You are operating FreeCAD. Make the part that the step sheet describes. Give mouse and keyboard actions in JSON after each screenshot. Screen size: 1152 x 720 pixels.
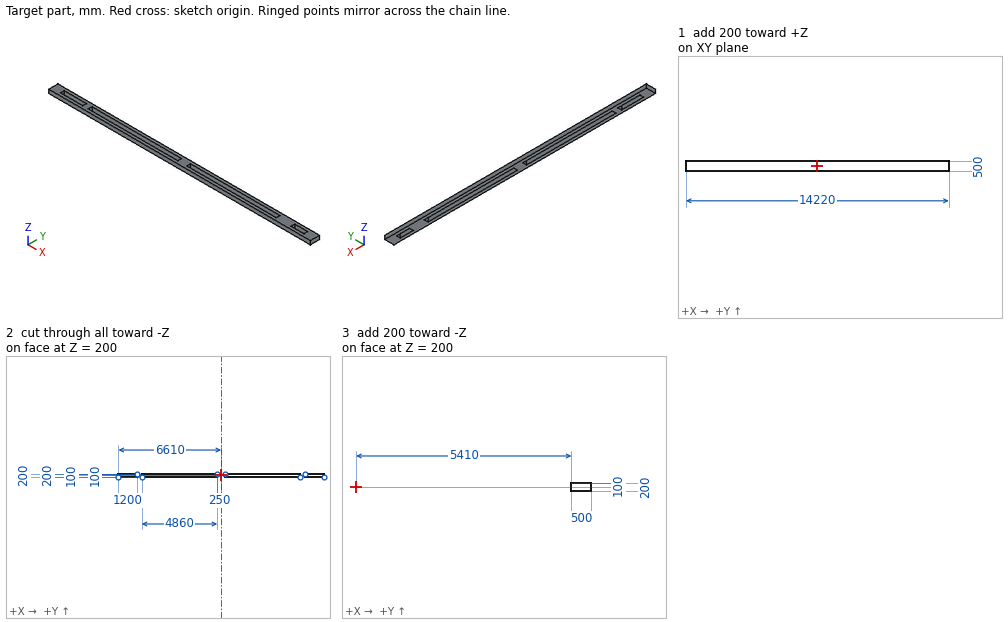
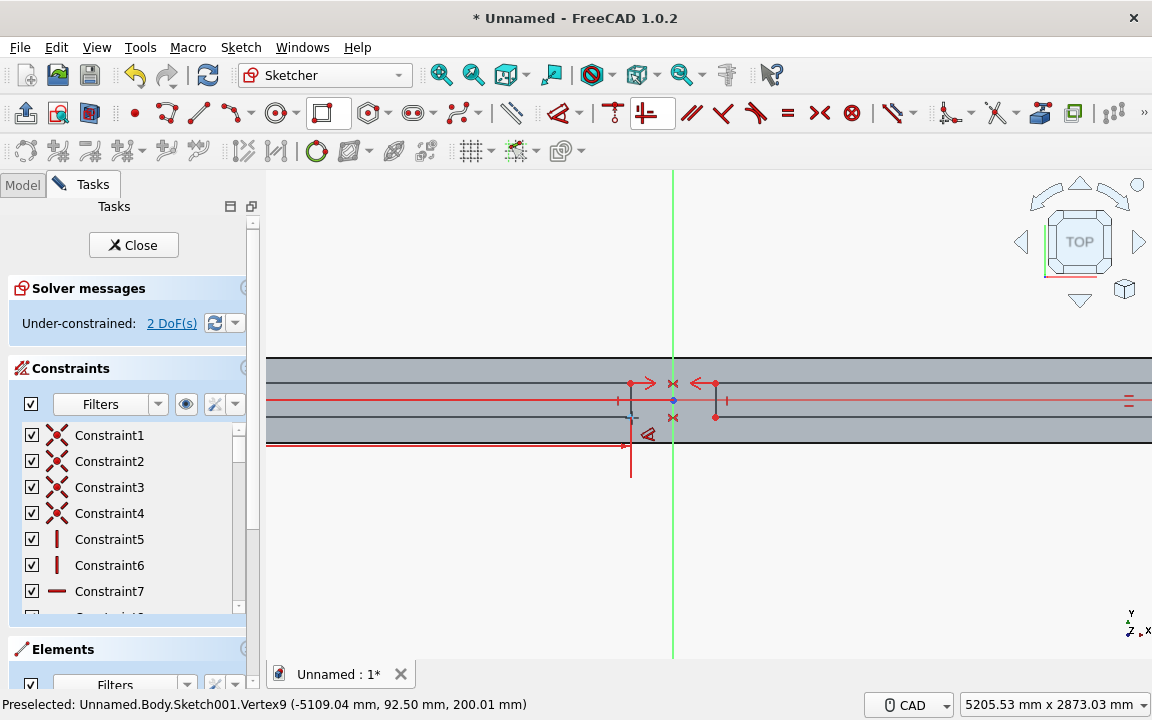
{"action": "left_click", "coordinate": [631, 417]}
{"action": "left_click", "coordinate": [652, 451]}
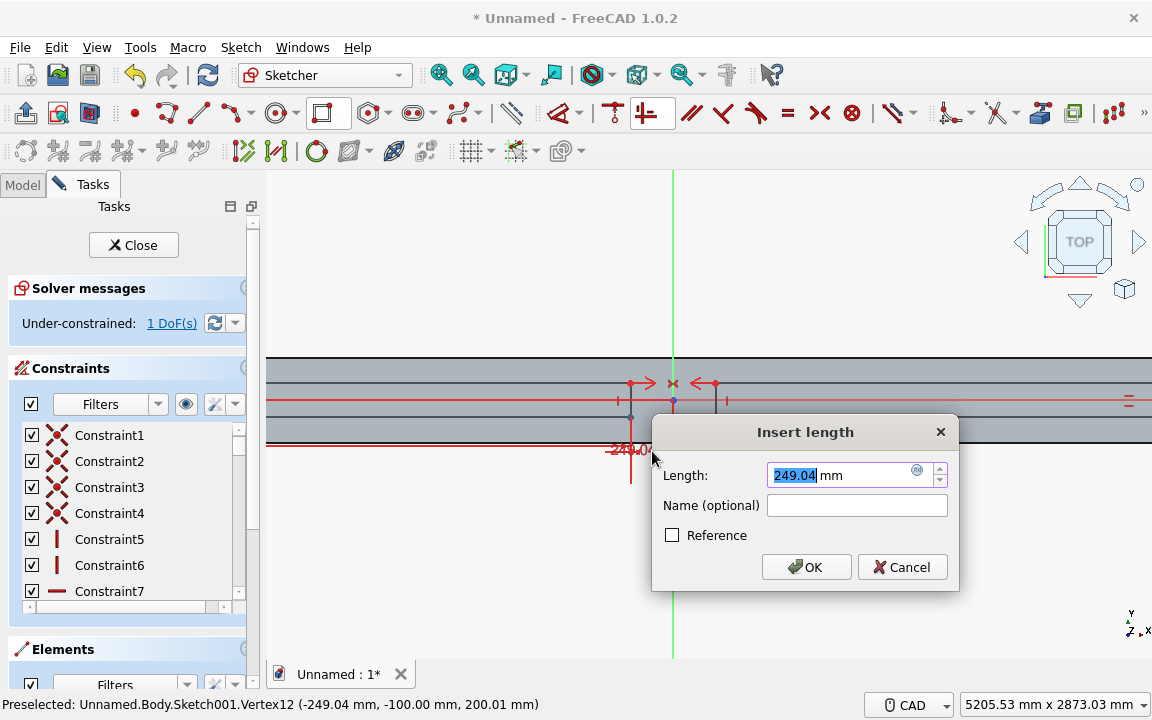
{"action": "type", "text": "250"}
{"action": "key", "text": "Return"}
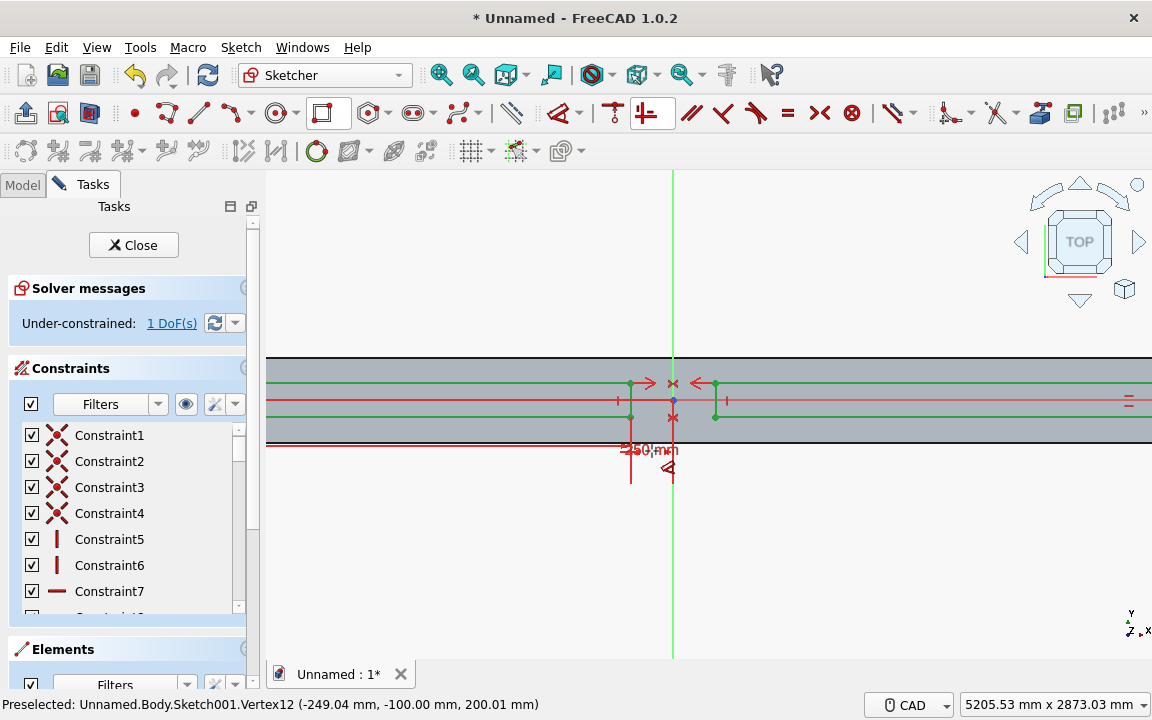
{"action": "scroll", "coordinate": [632, 418], "scroll_direction": "down", "scroll_amount": 8}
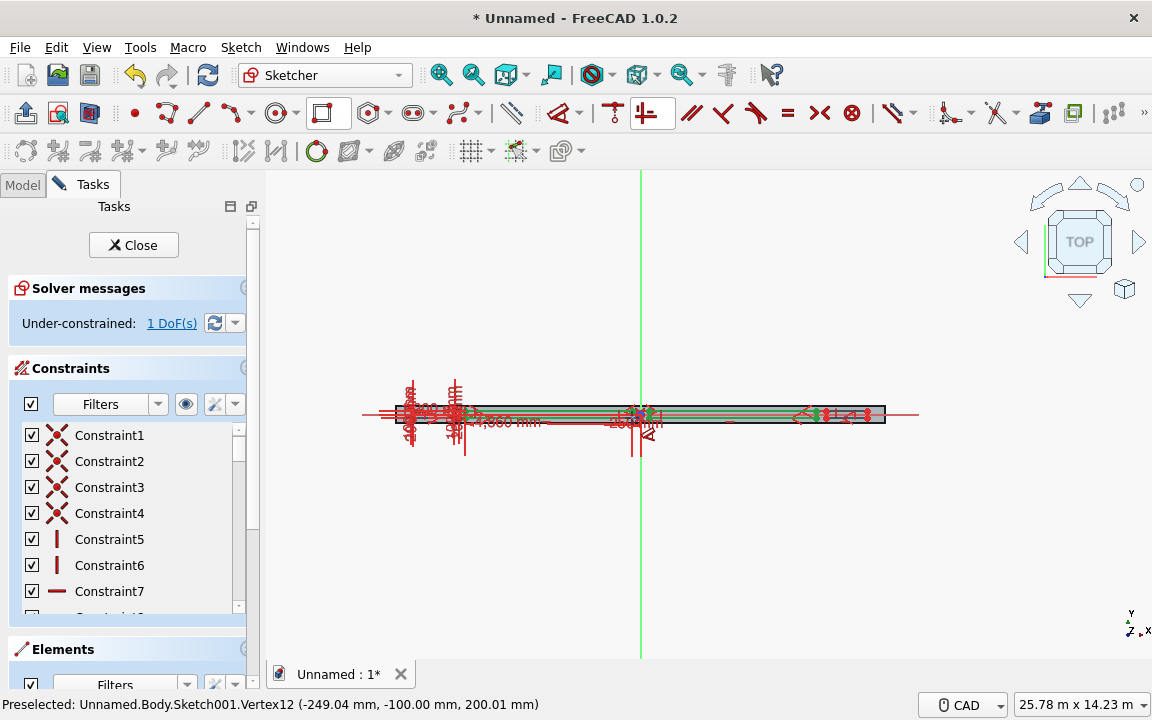
{"action": "scroll", "coordinate": [413, 411], "scroll_direction": "up", "scroll_amount": 3}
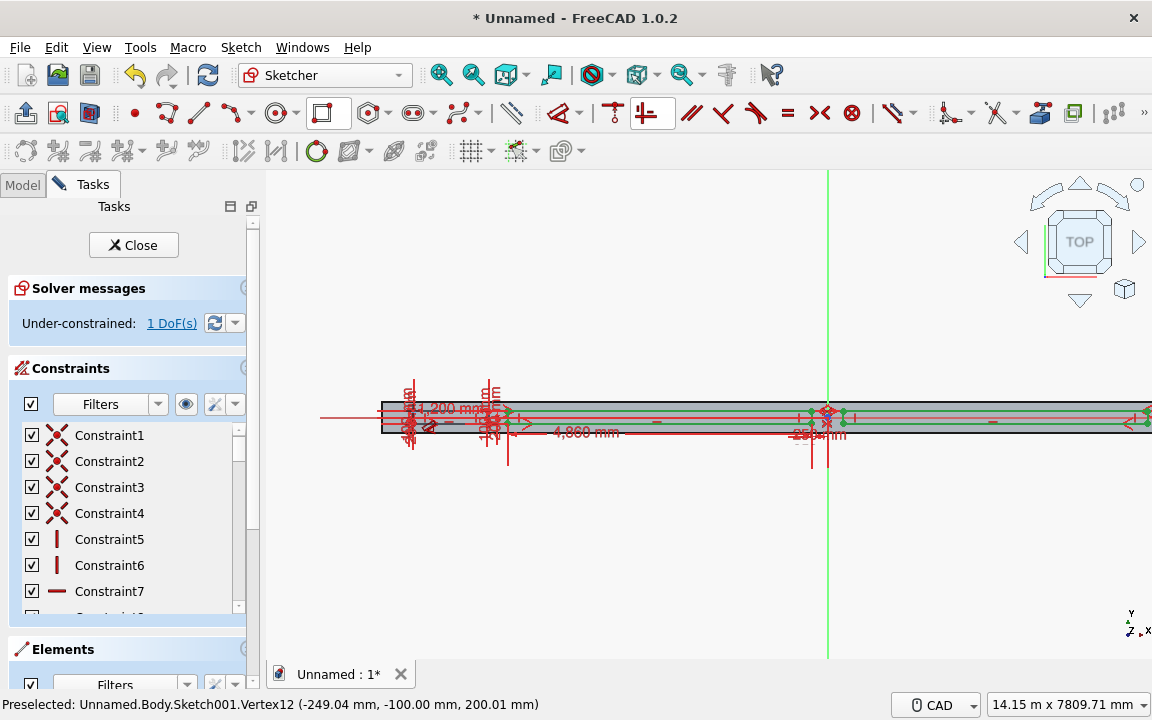
{"action": "left_click", "coordinate": [414, 411]}
{"action": "left_click", "coordinate": [621, 377]}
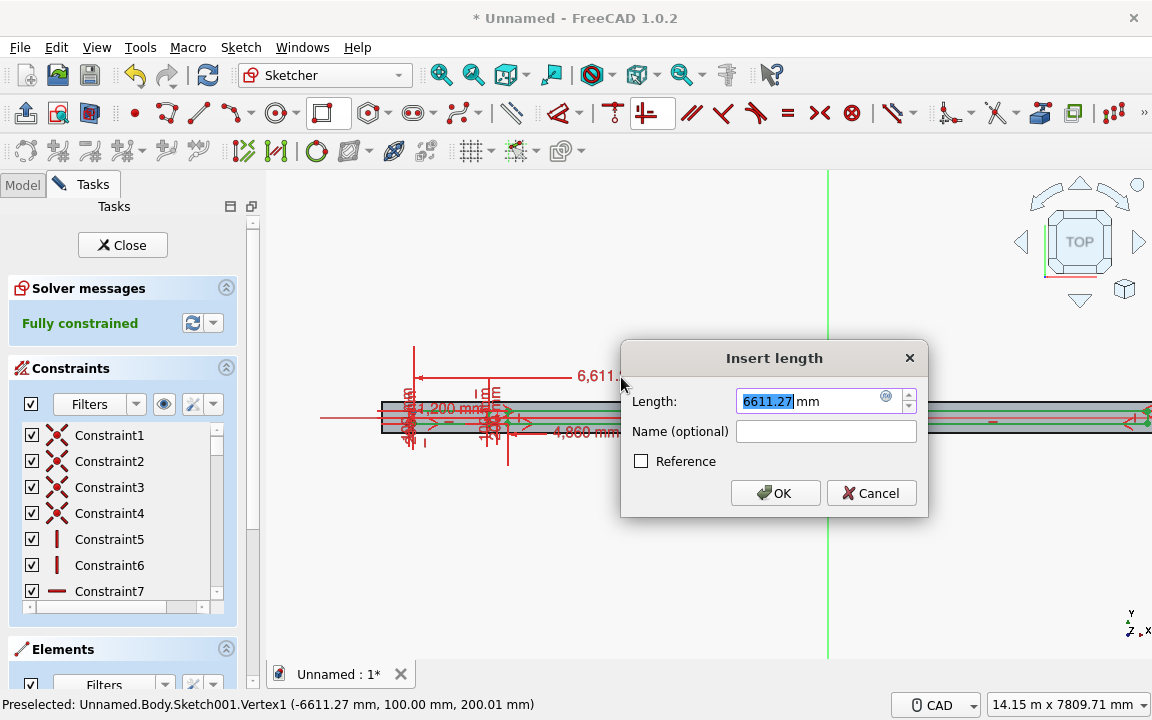
{"action": "type", "text": "6610"}
{"action": "key", "text": "Return"}
{"action": "key", "text": "Escape"}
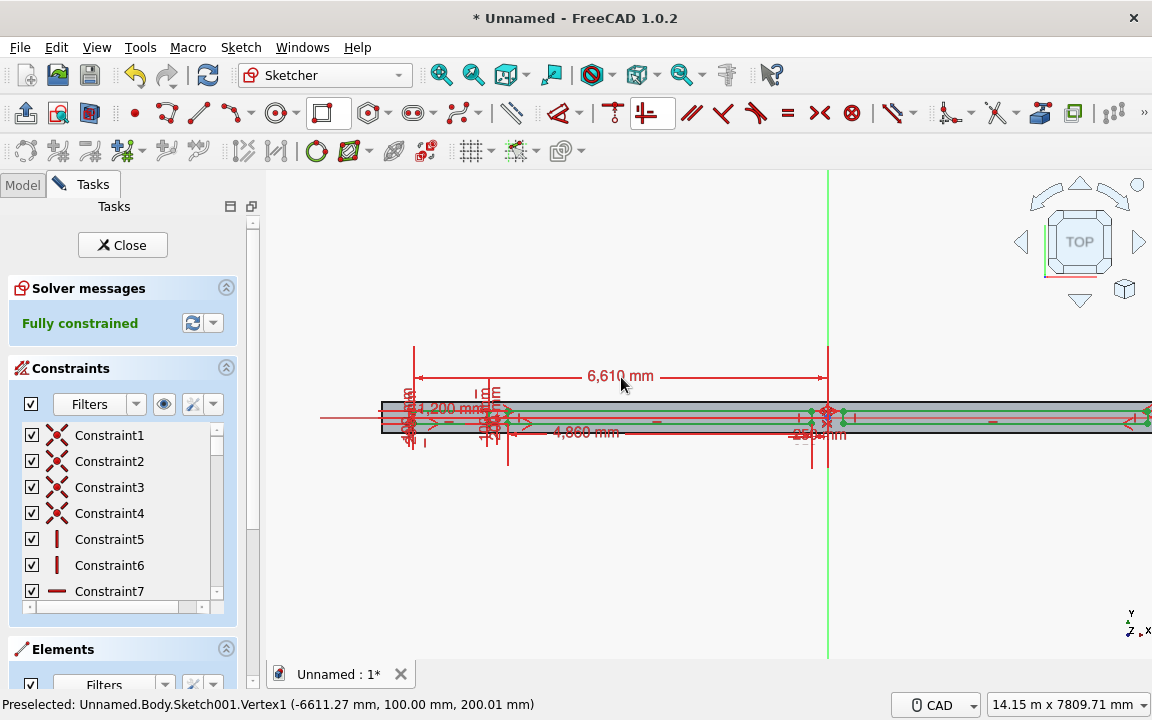
{"action": "left_click", "coordinate": [123, 245]}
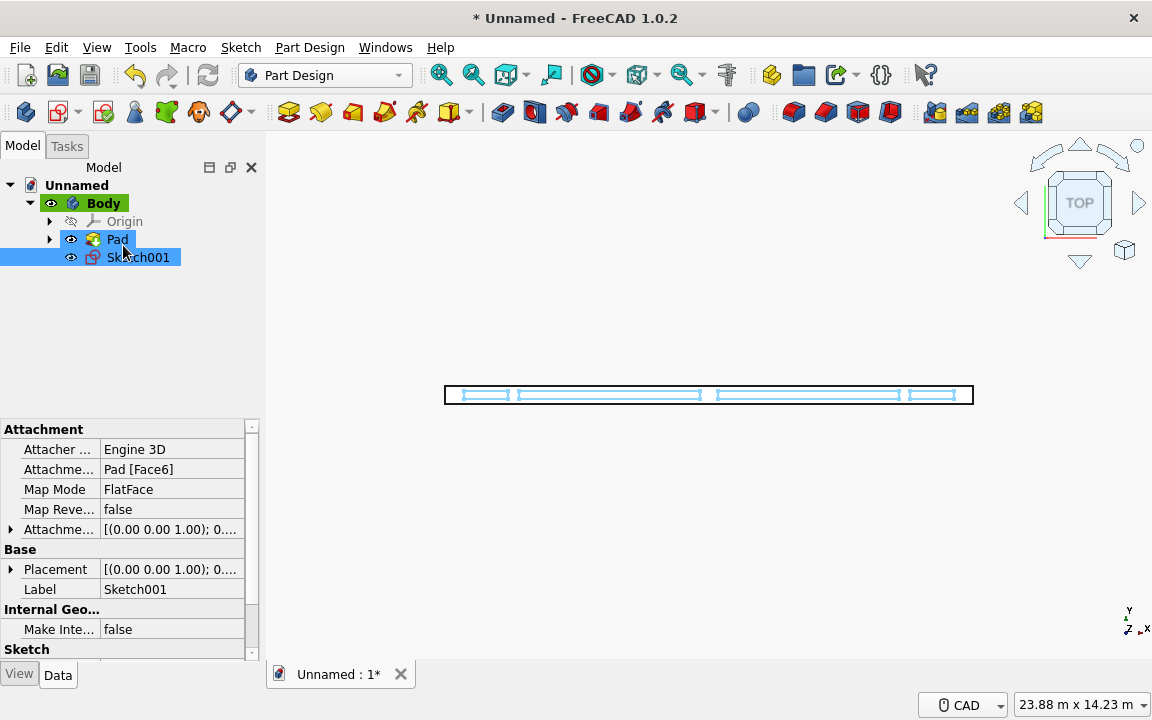
{"action": "left_click", "coordinate": [504, 112]}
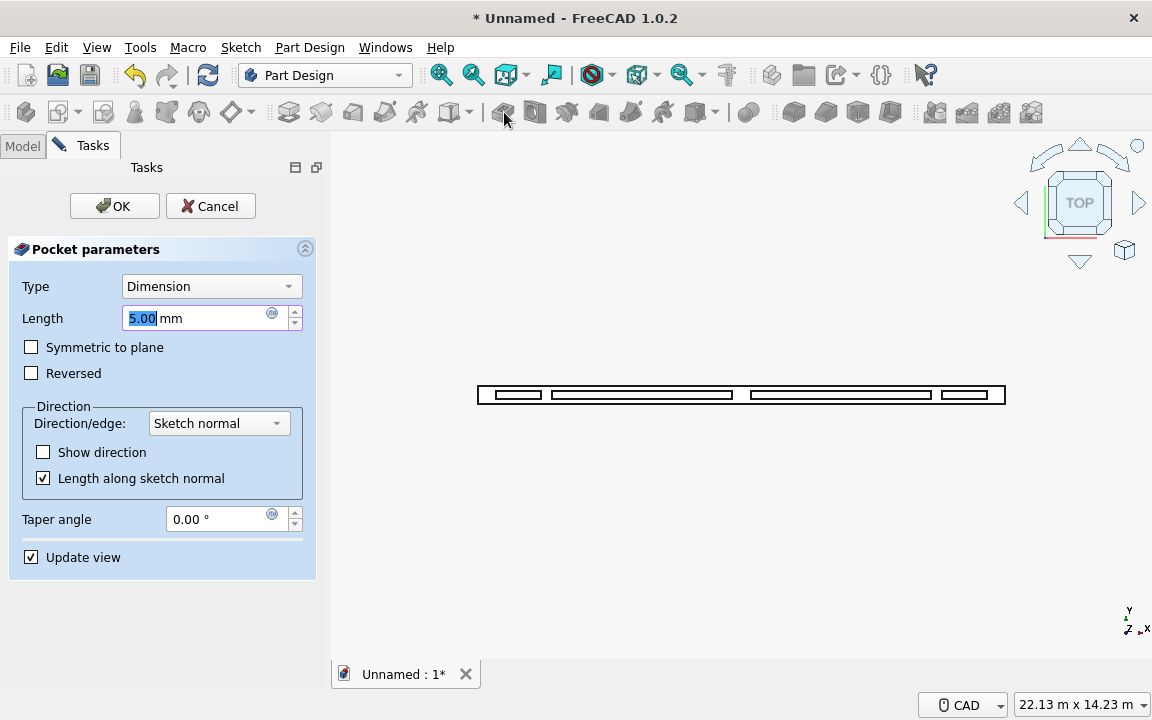
{"action": "left_click", "coordinate": [212, 286]}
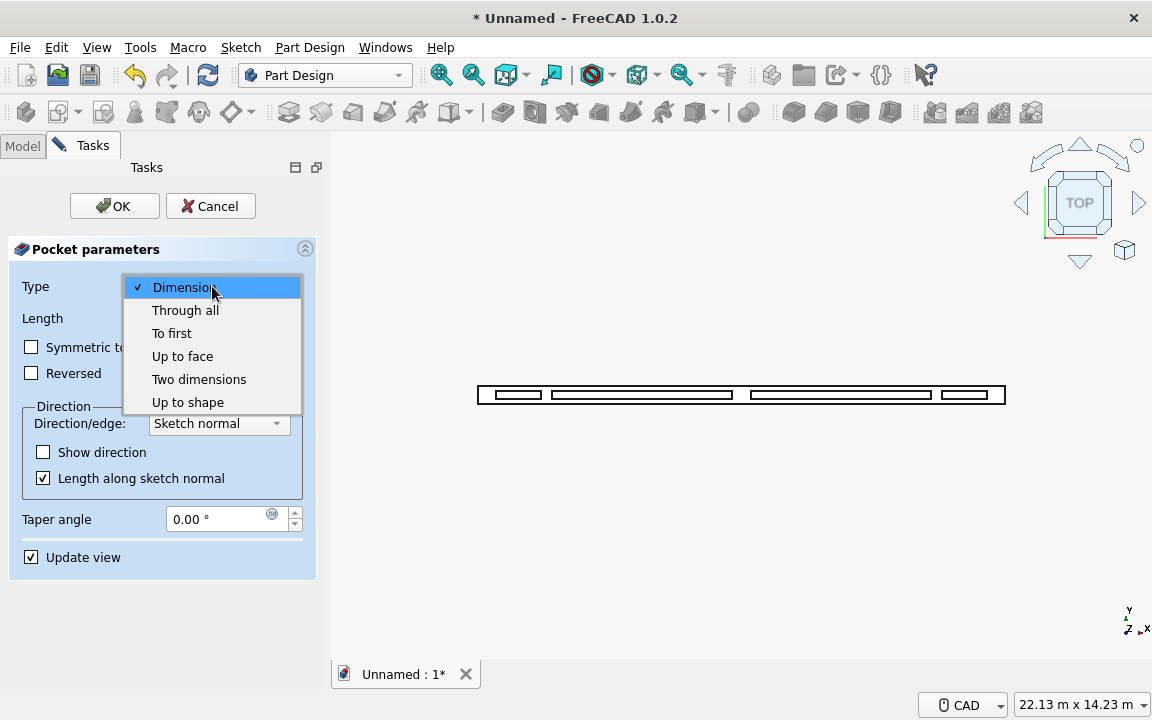
{"action": "left_click", "coordinate": [212, 310]}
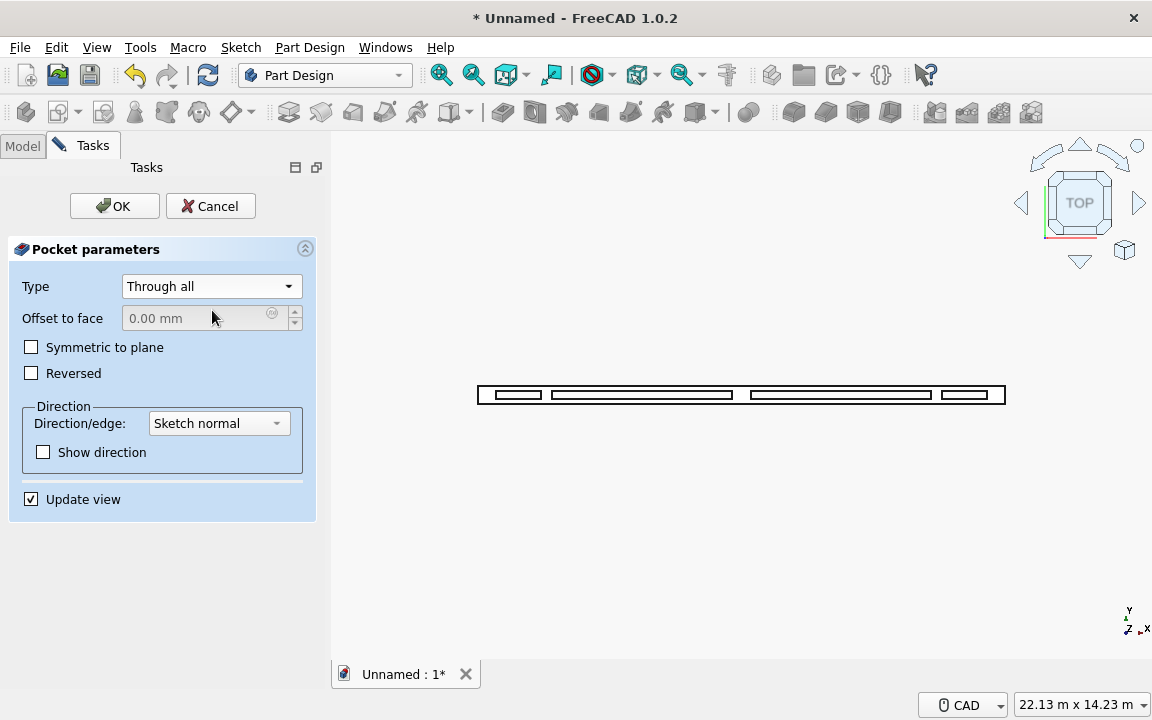
{"action": "left_click", "coordinate": [115, 206]}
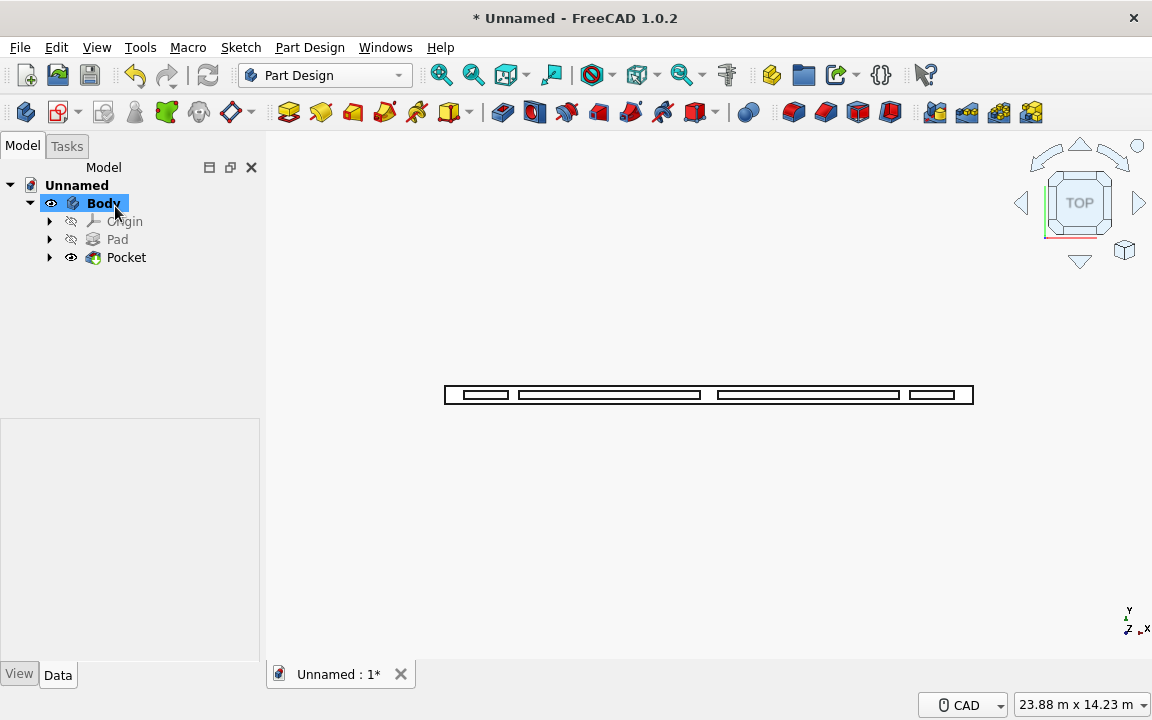
{"action": "left_click", "coordinate": [709, 394]}